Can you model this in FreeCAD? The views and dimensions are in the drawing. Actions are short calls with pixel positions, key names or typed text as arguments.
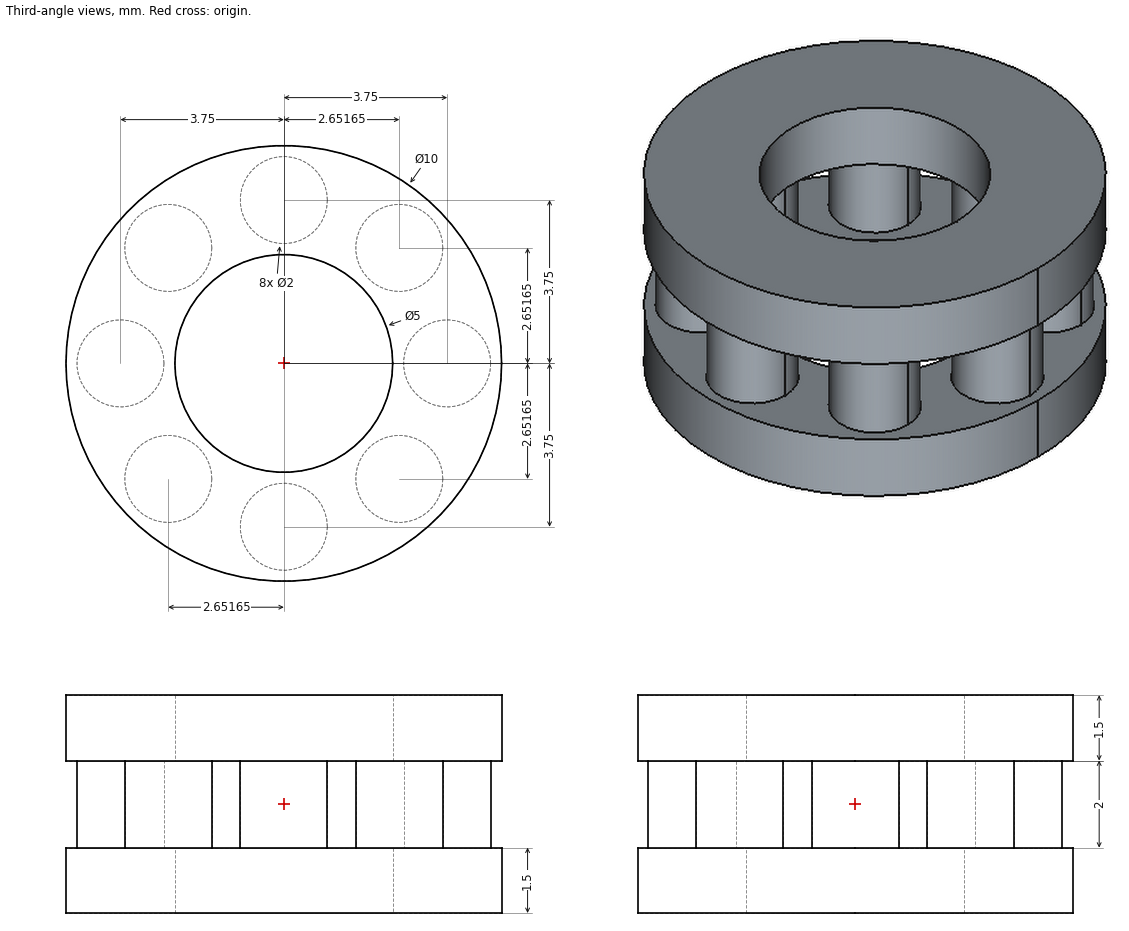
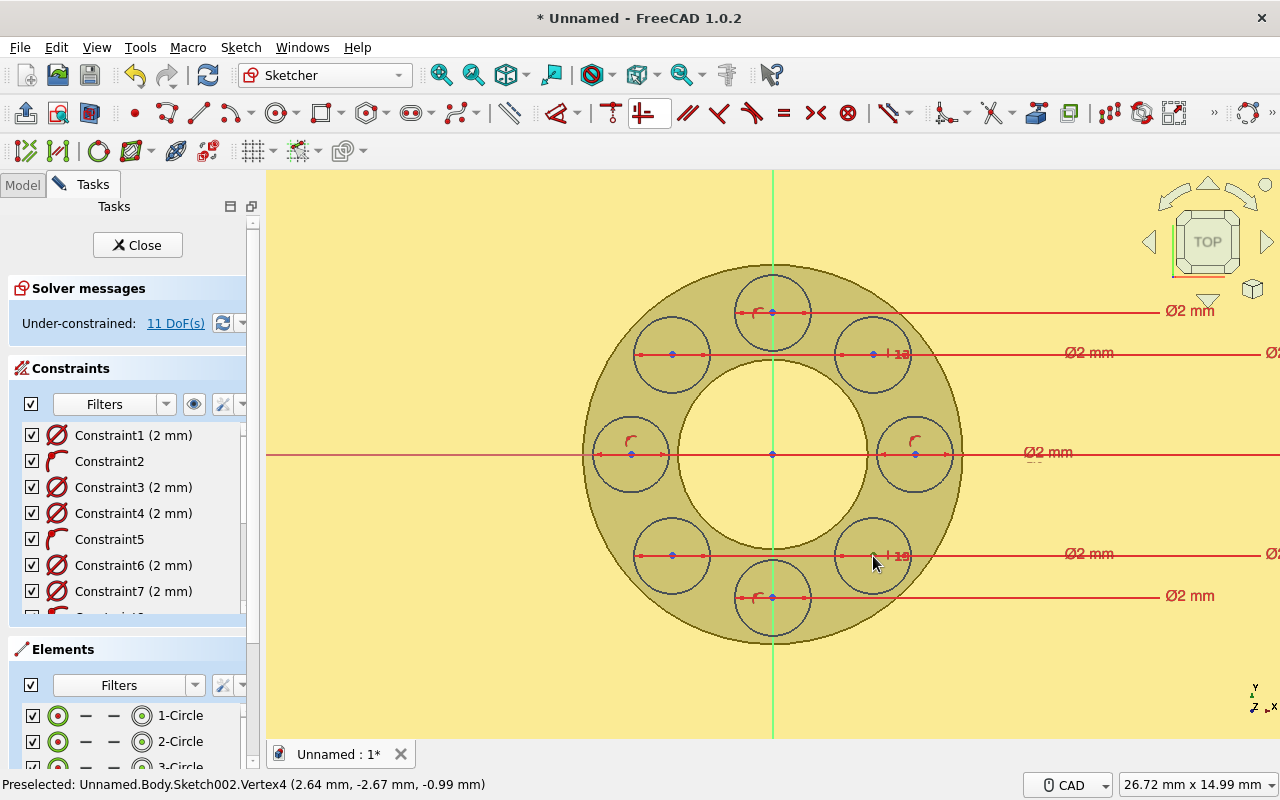
click(672, 556)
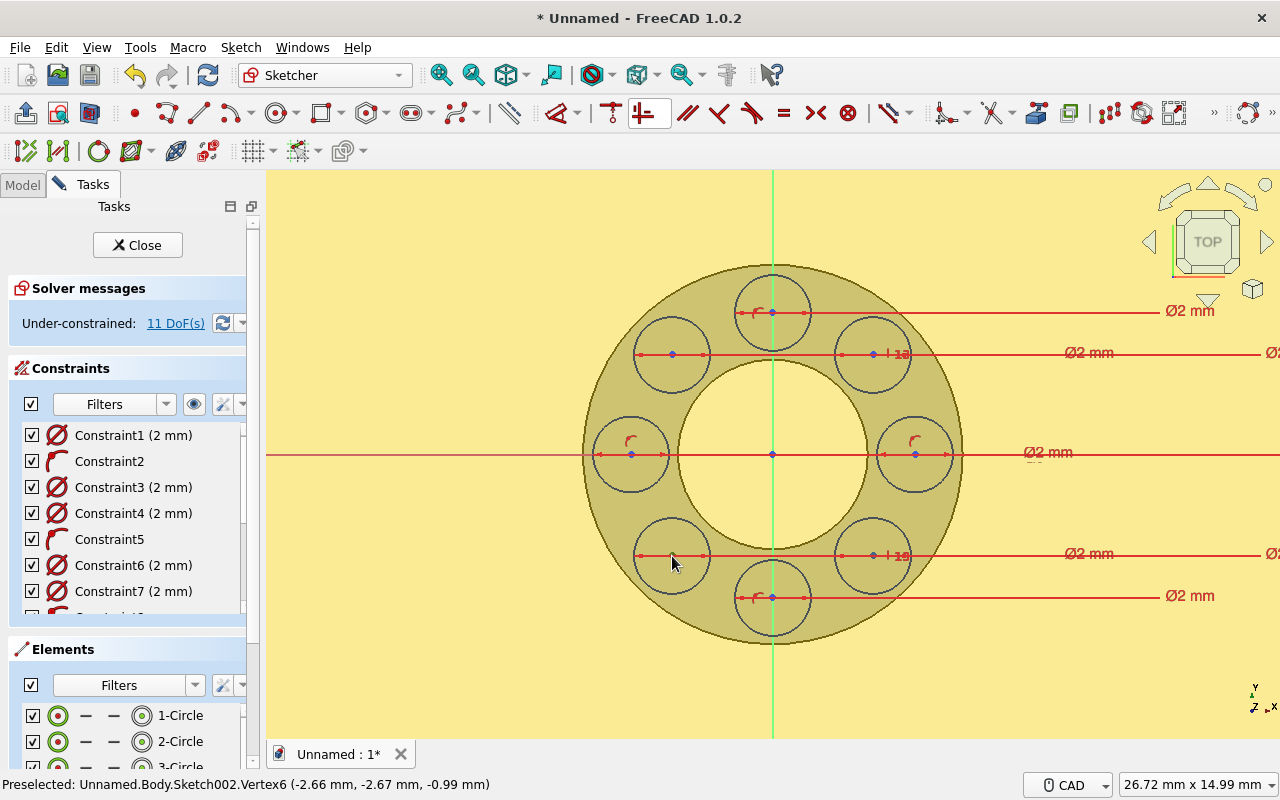
key(h)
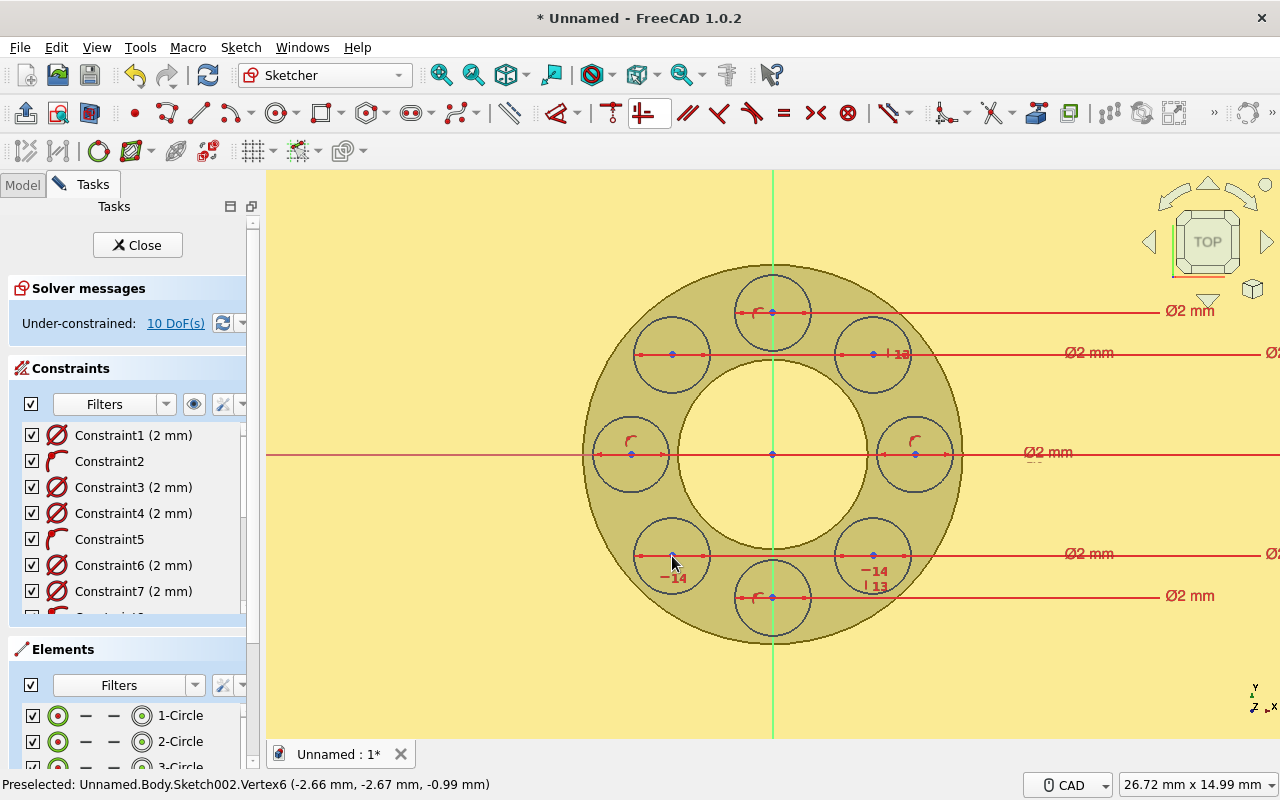
click(672, 556)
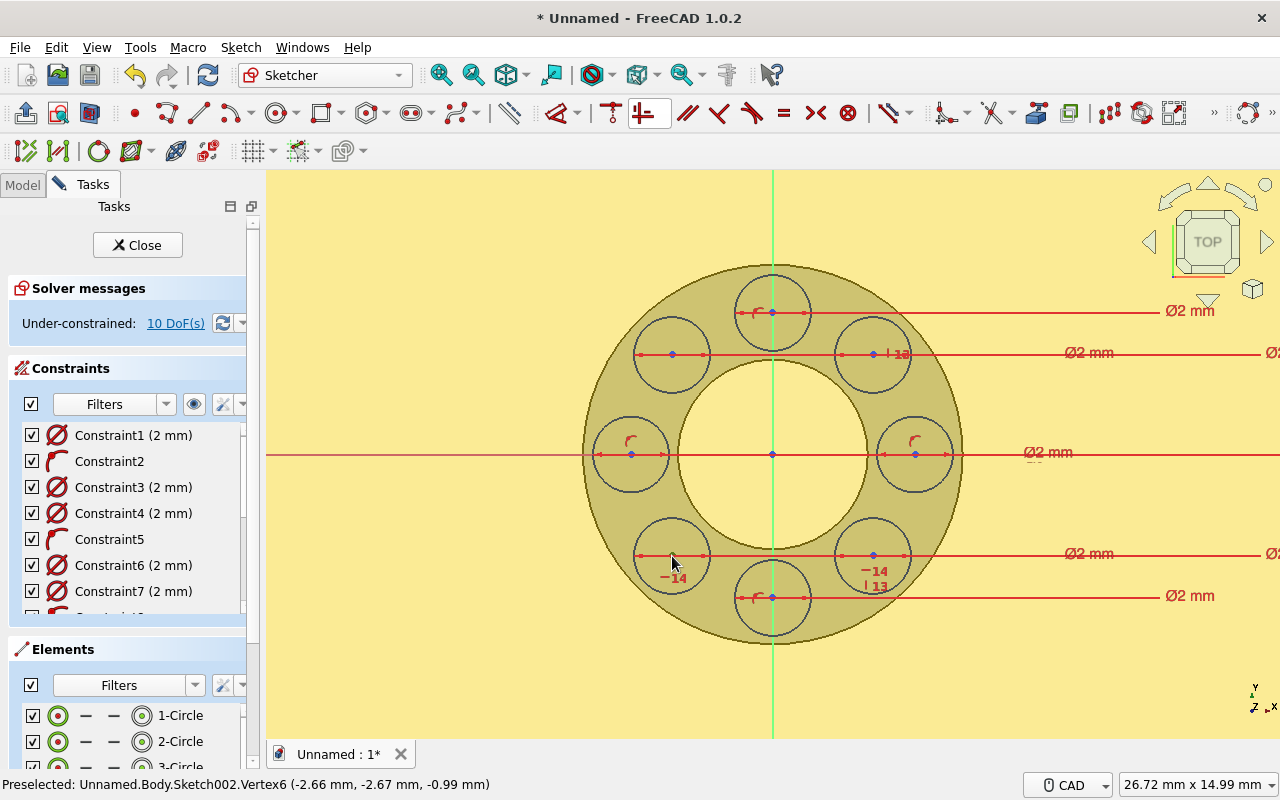
click(672, 355)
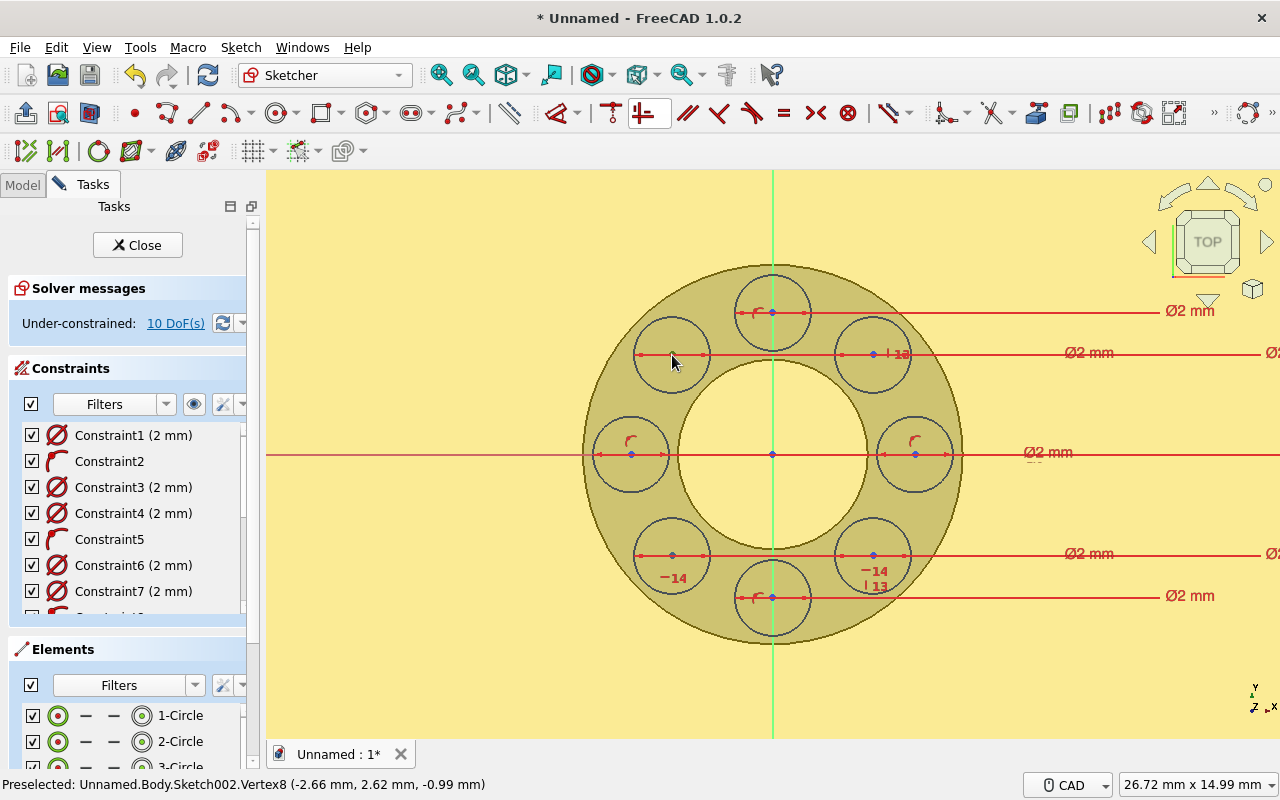
key(v)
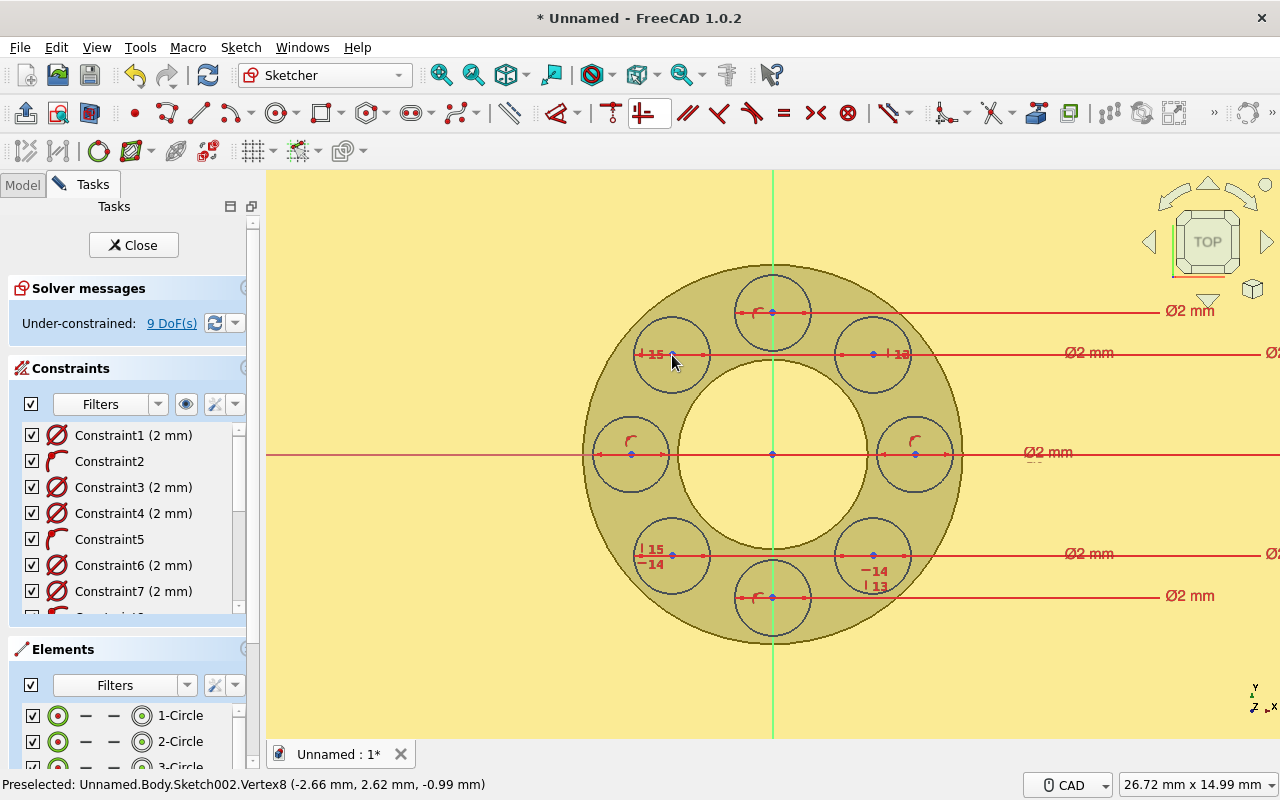
click(873, 355)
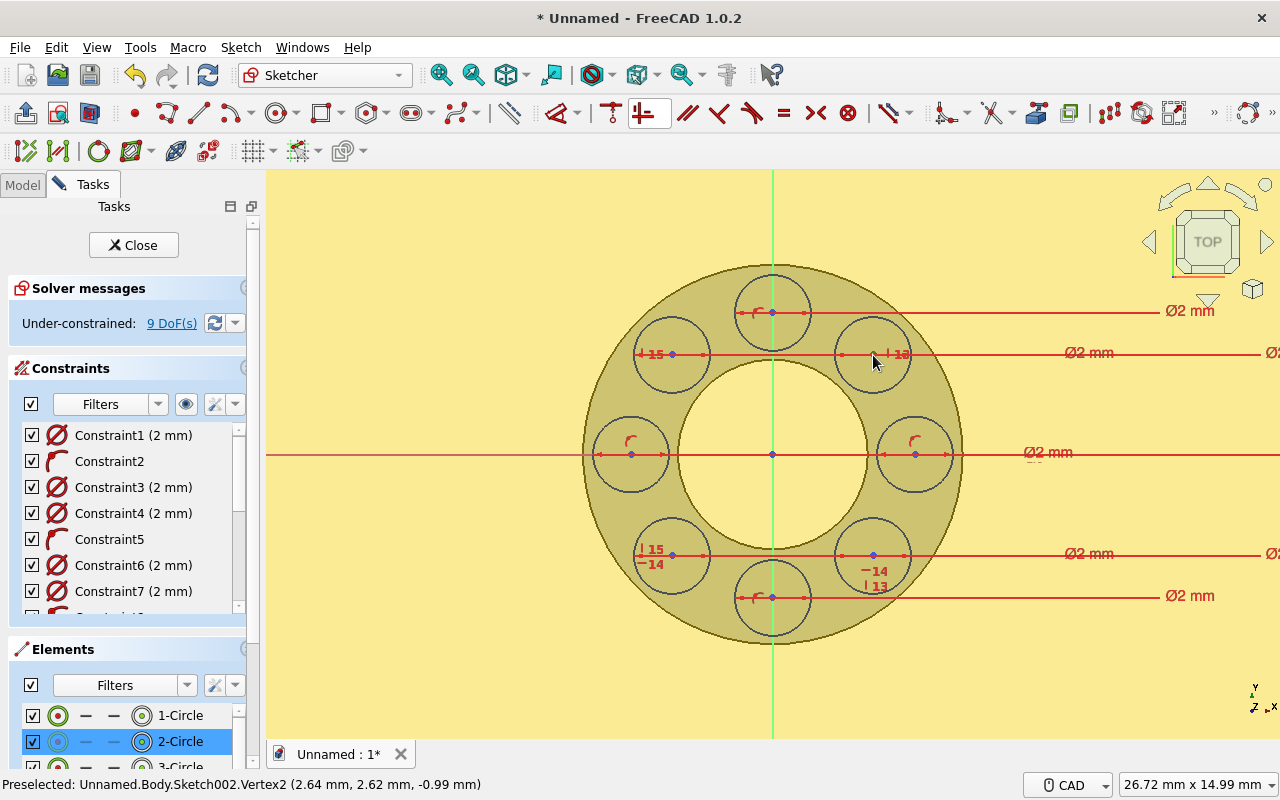
click(672, 355)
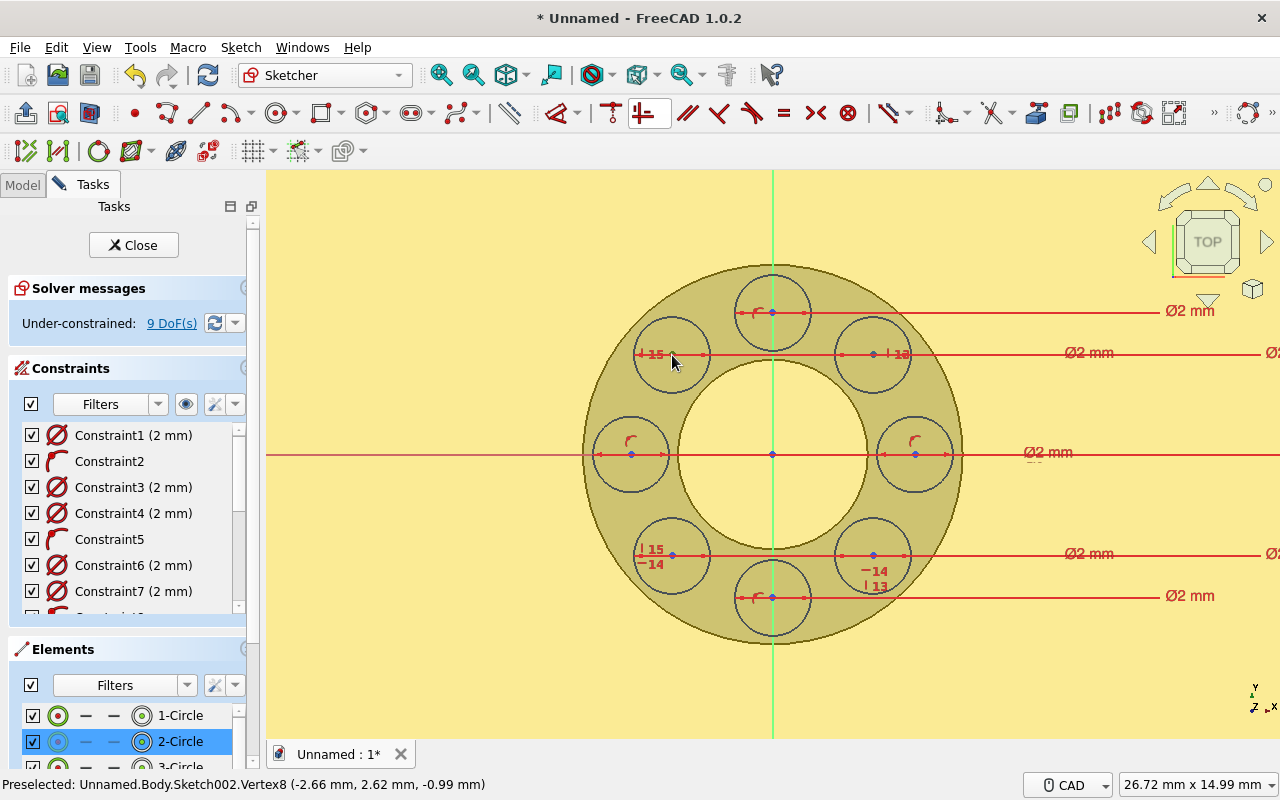
click(666, 114)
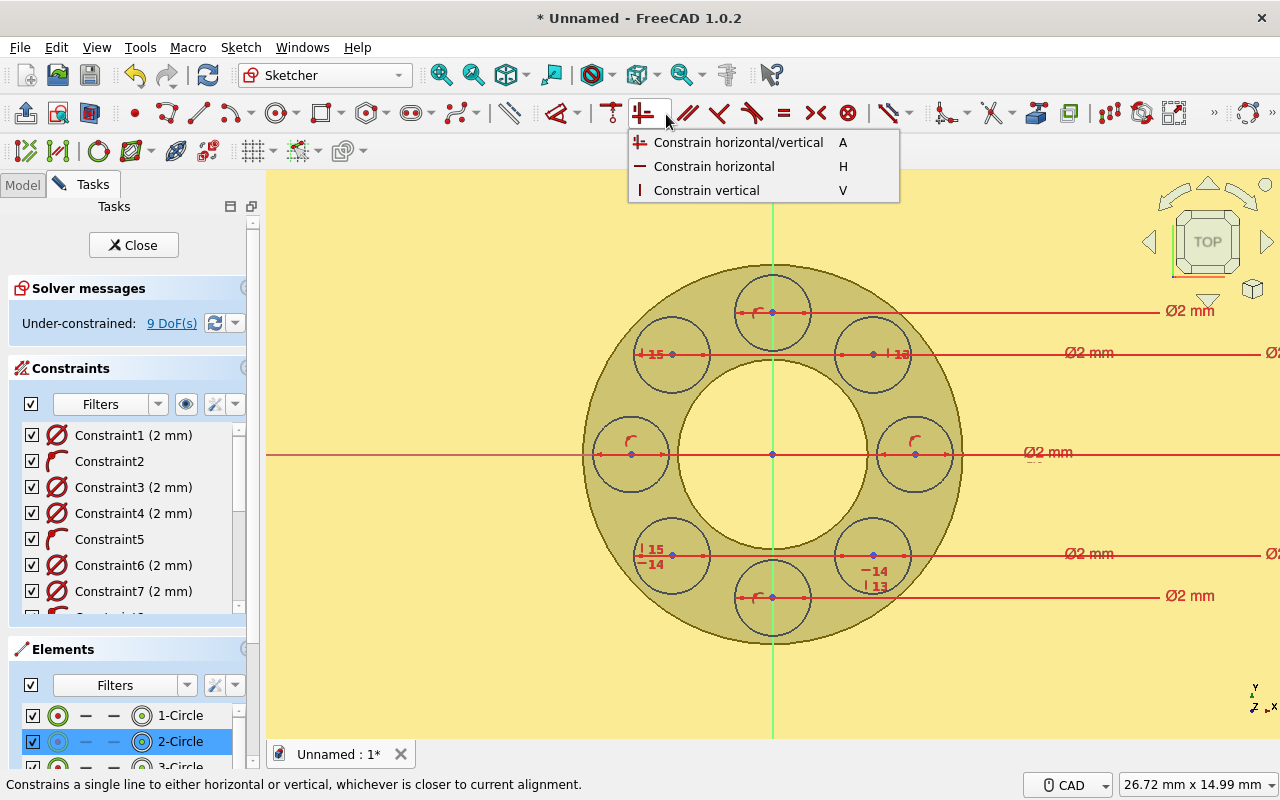
click(764, 166)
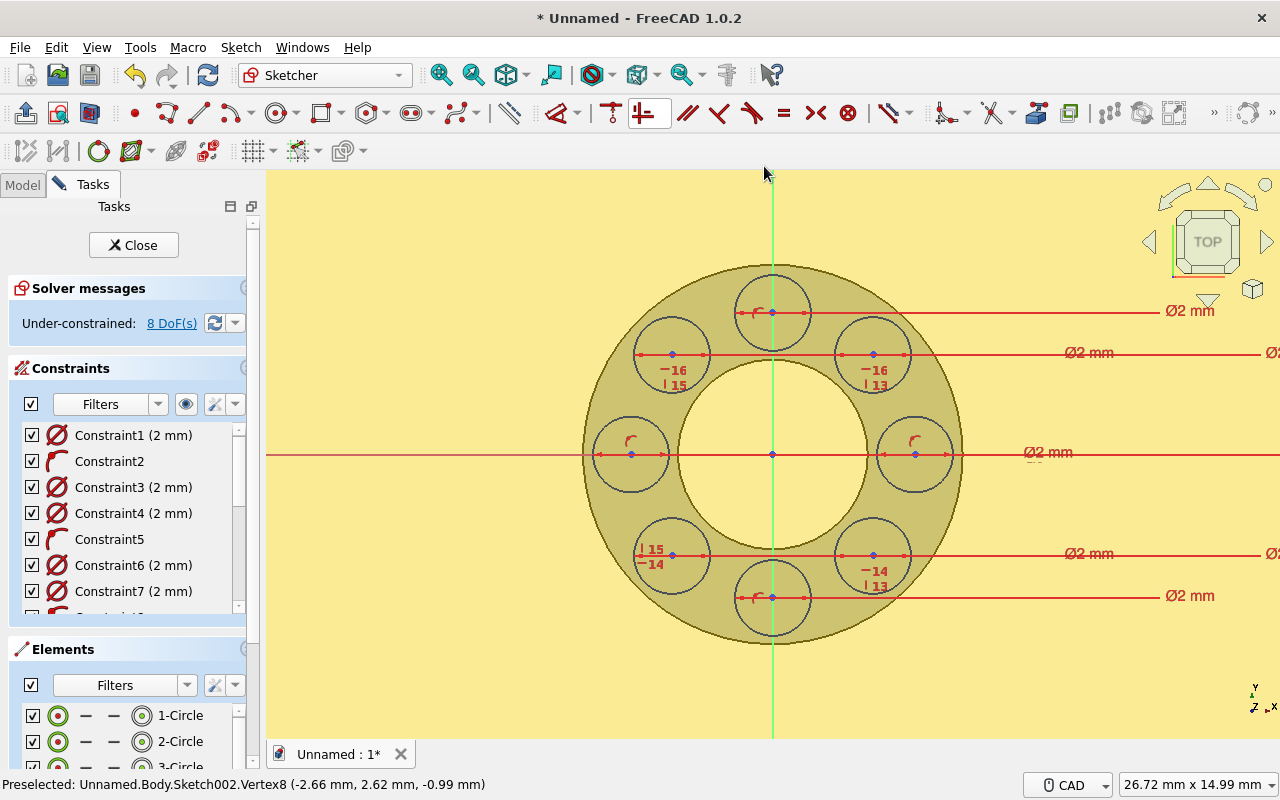
click(556, 114)